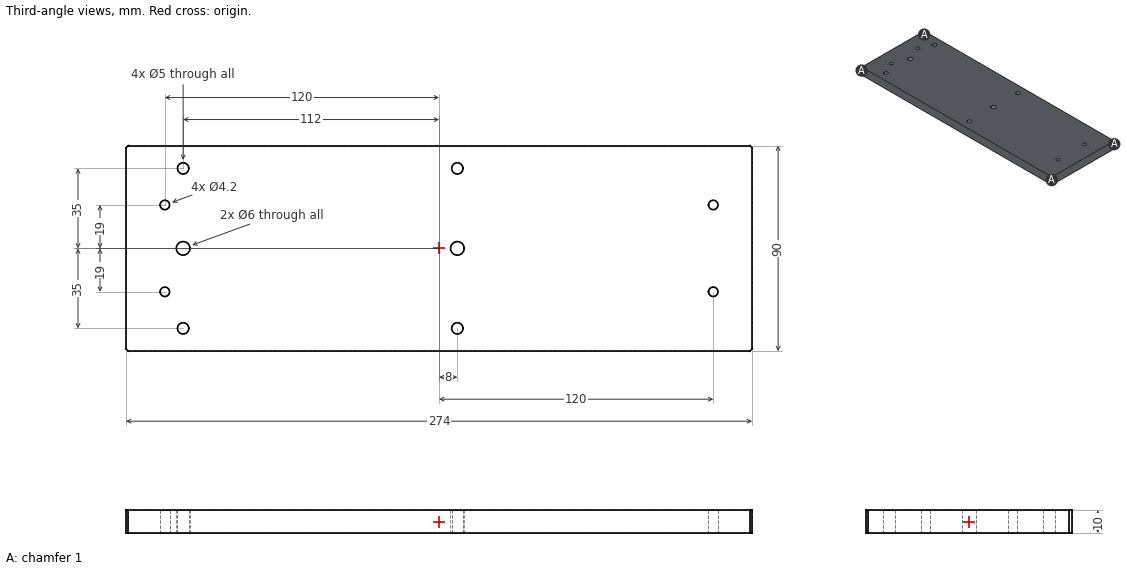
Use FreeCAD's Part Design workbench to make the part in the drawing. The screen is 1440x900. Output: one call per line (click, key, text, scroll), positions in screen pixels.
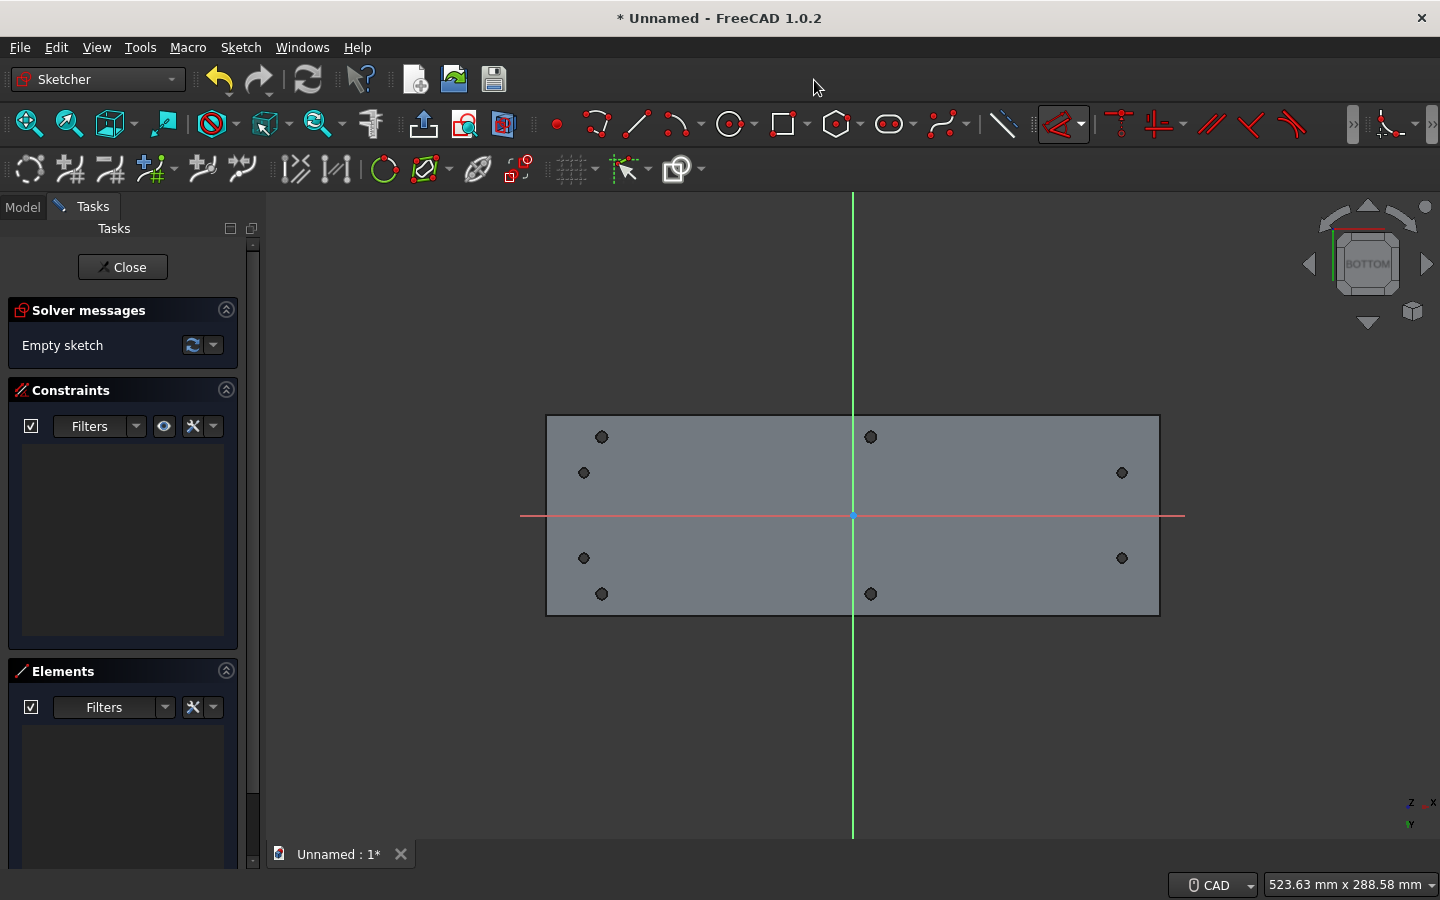
scroll(697, 516, up, 4)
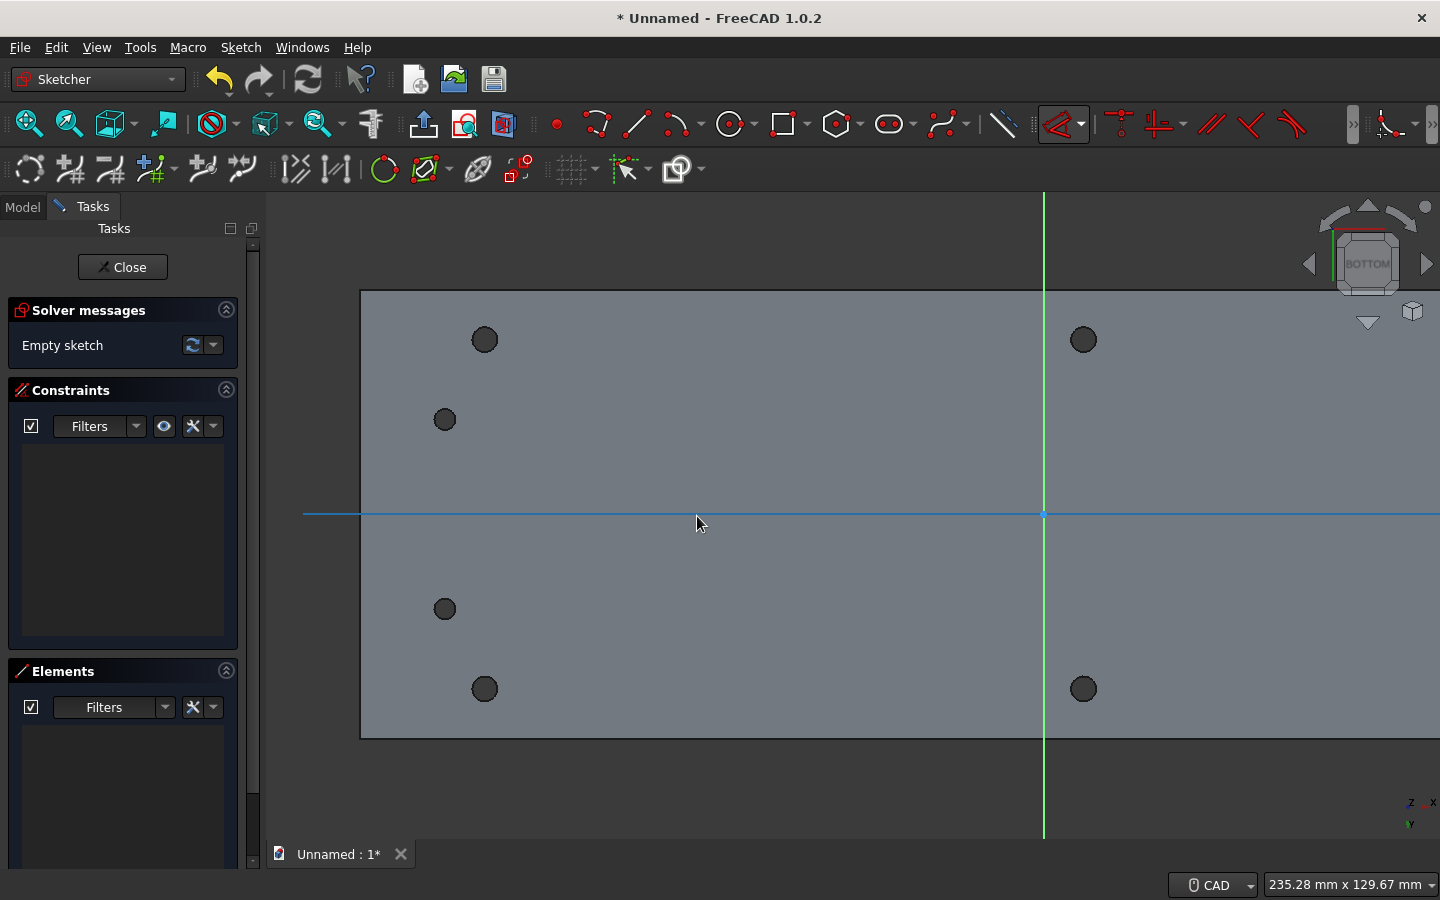
key(g)
key(c)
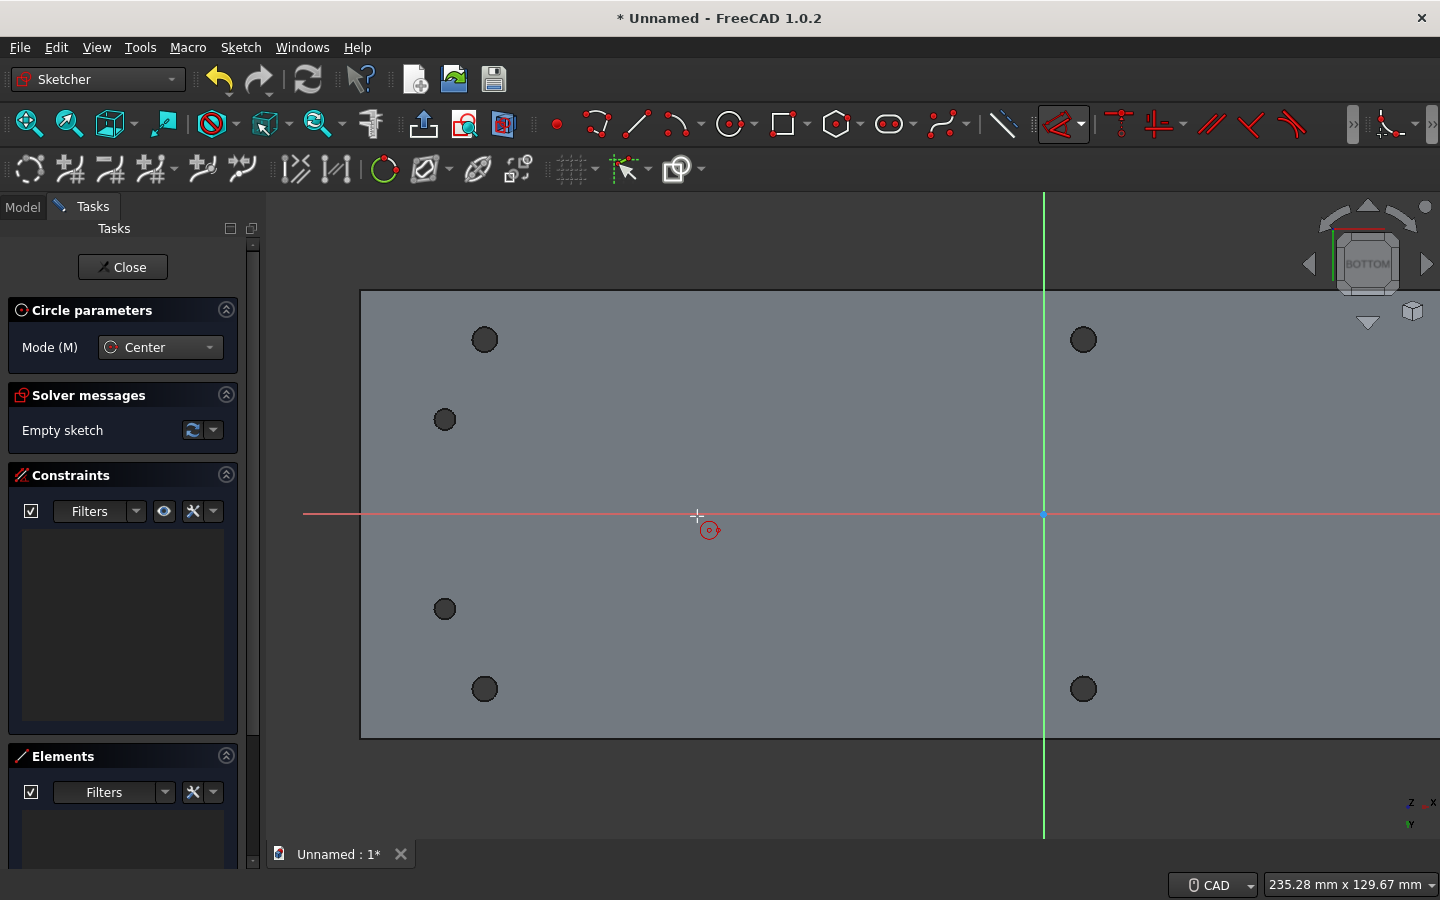
scroll(485, 514, up, 3)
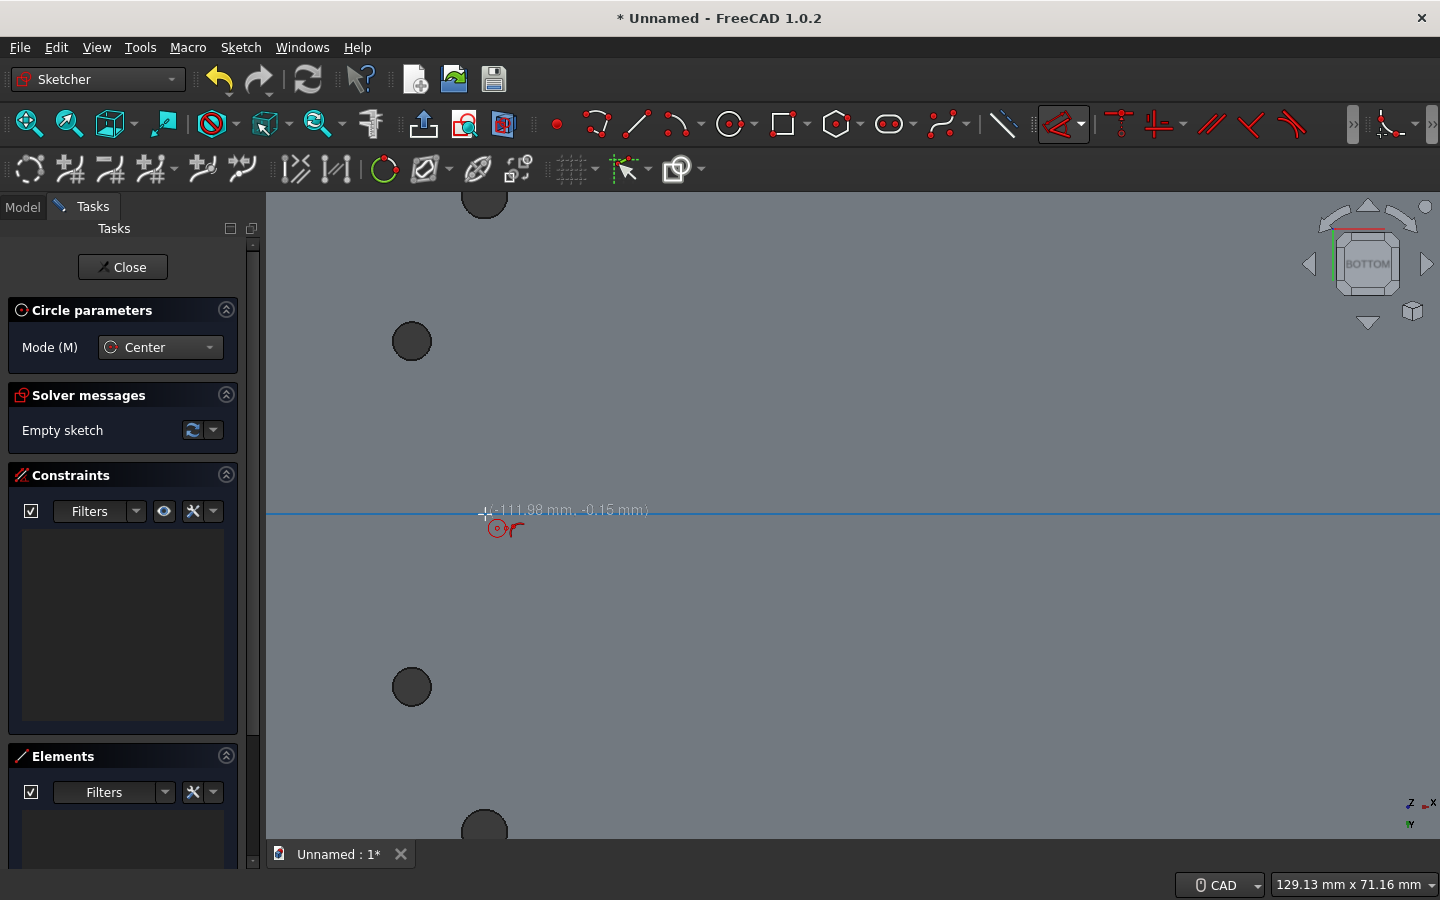
click(485, 514)
click(504, 495)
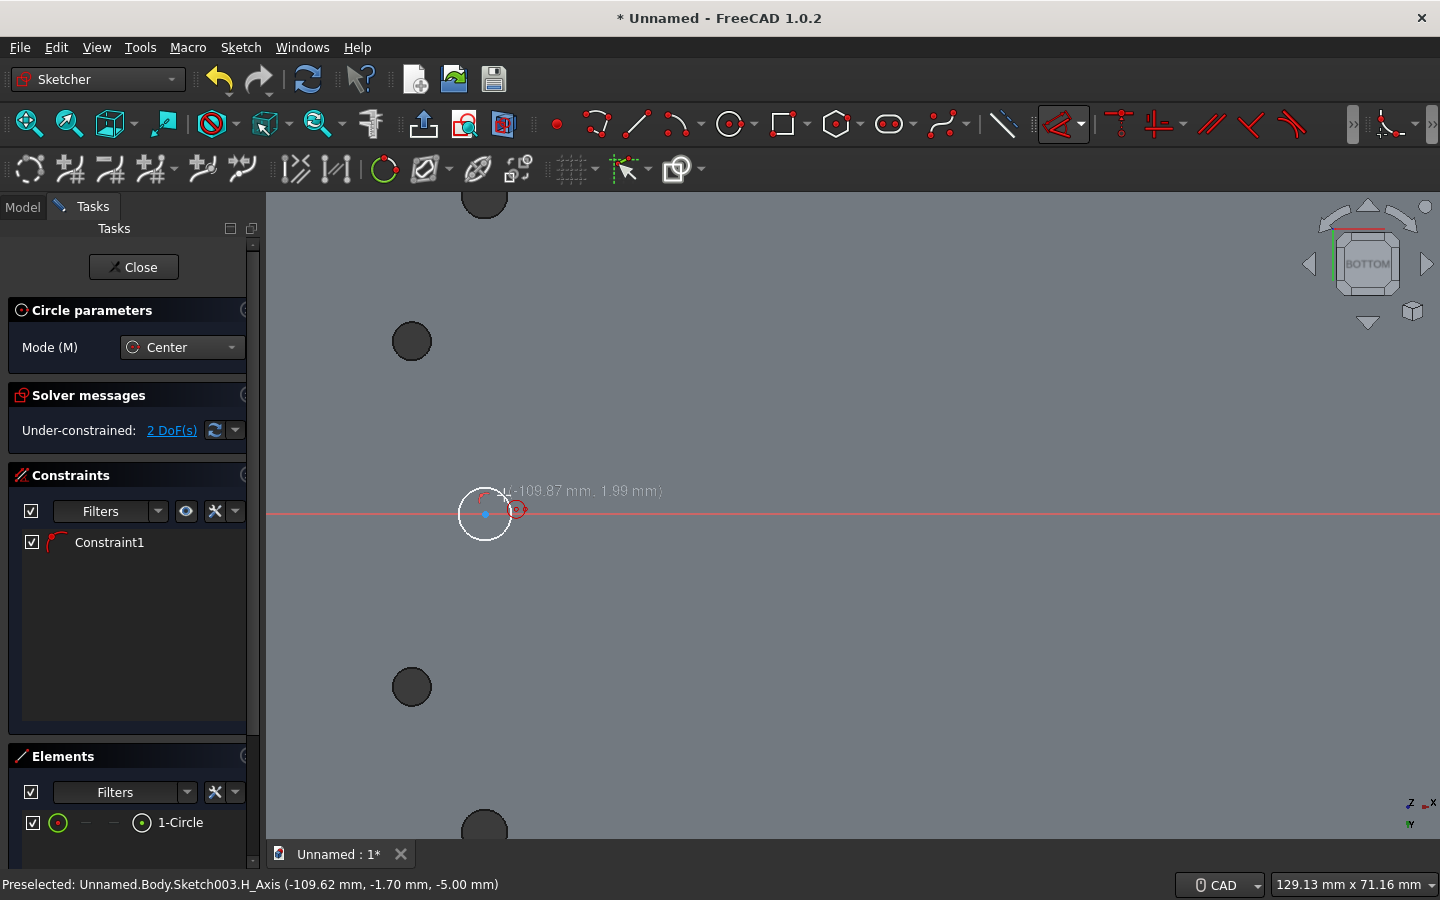
scroll(486, 517, down, 3)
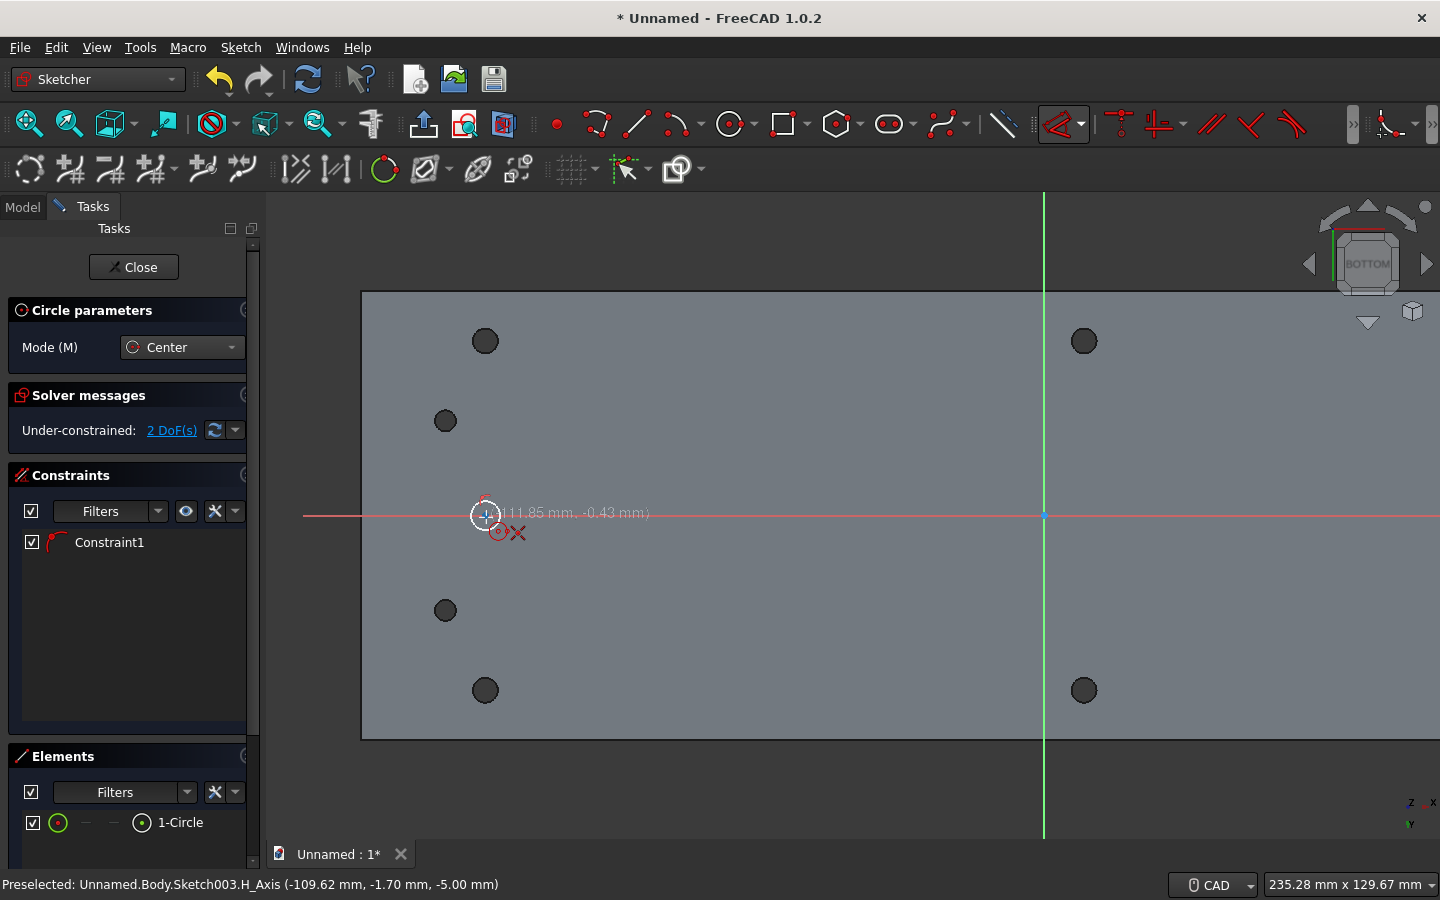
scroll(1084, 516, up, 3)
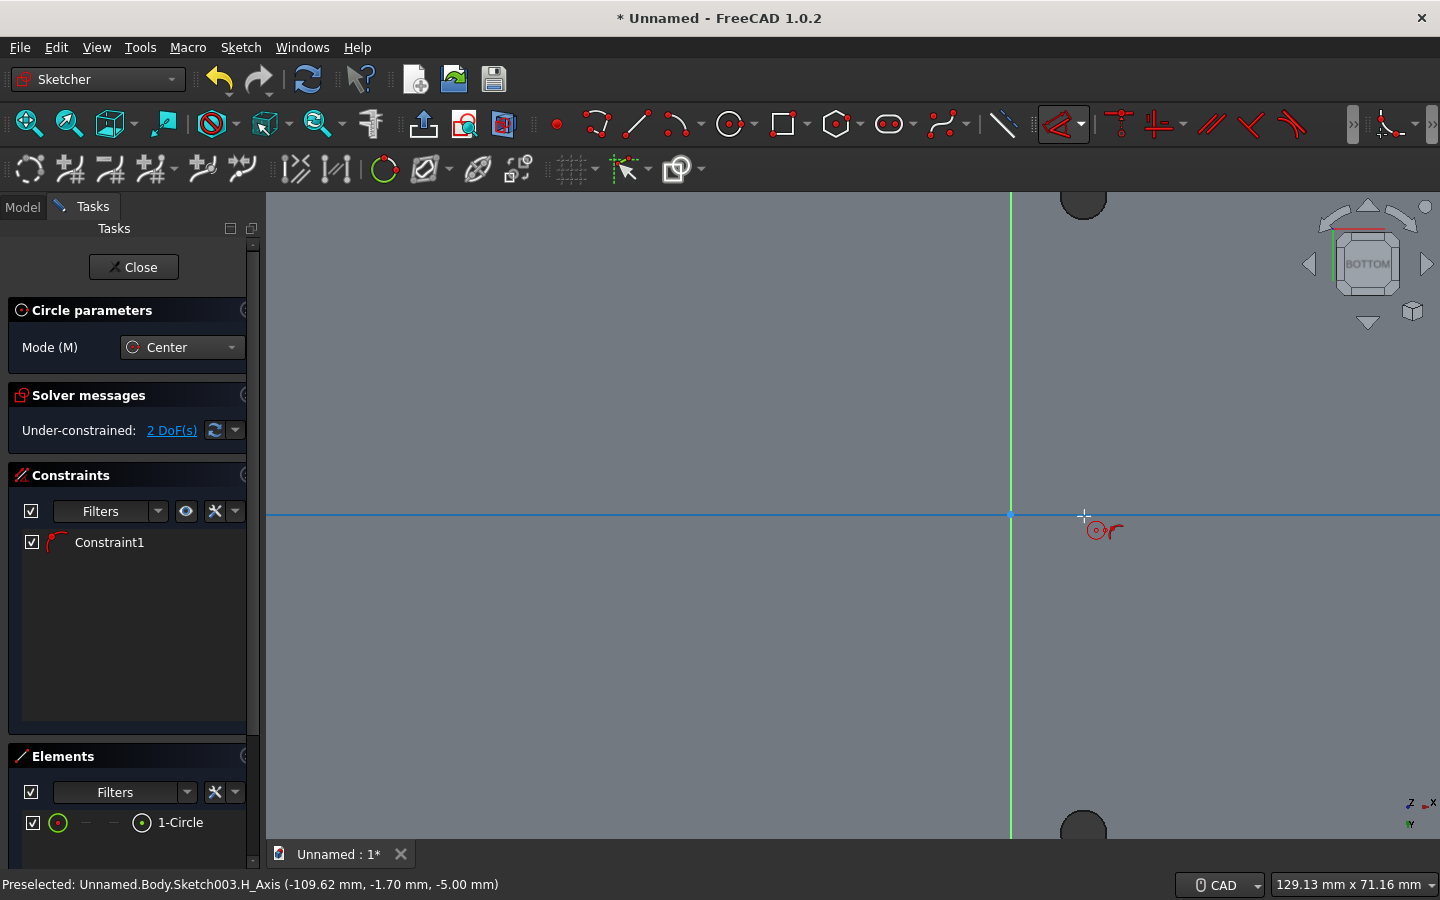
click(1084, 515)
click(1103, 496)
key(Escape)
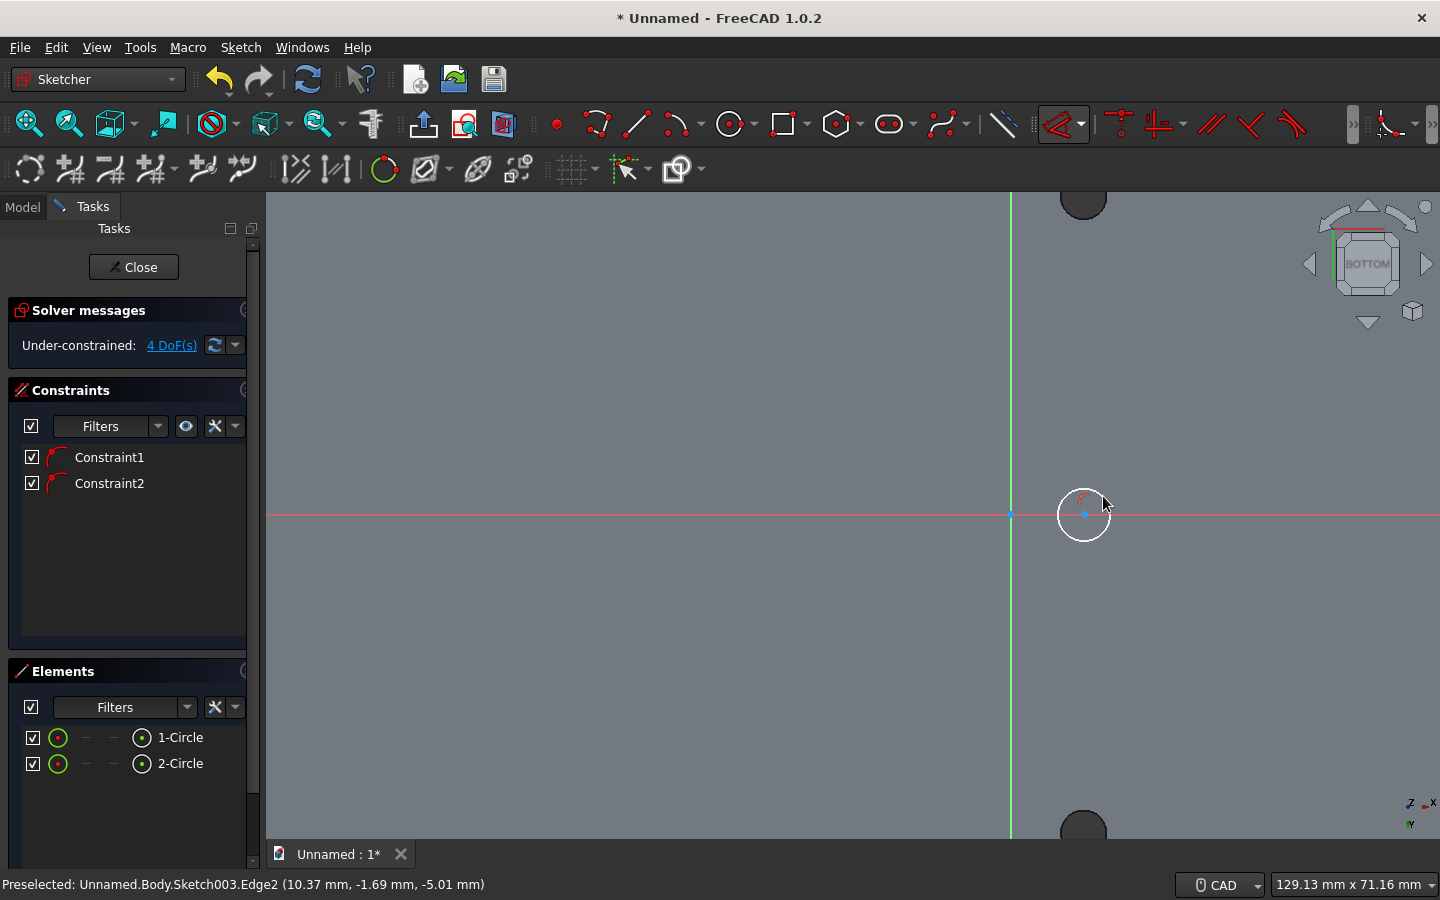
scroll(1084, 516, down, 3)